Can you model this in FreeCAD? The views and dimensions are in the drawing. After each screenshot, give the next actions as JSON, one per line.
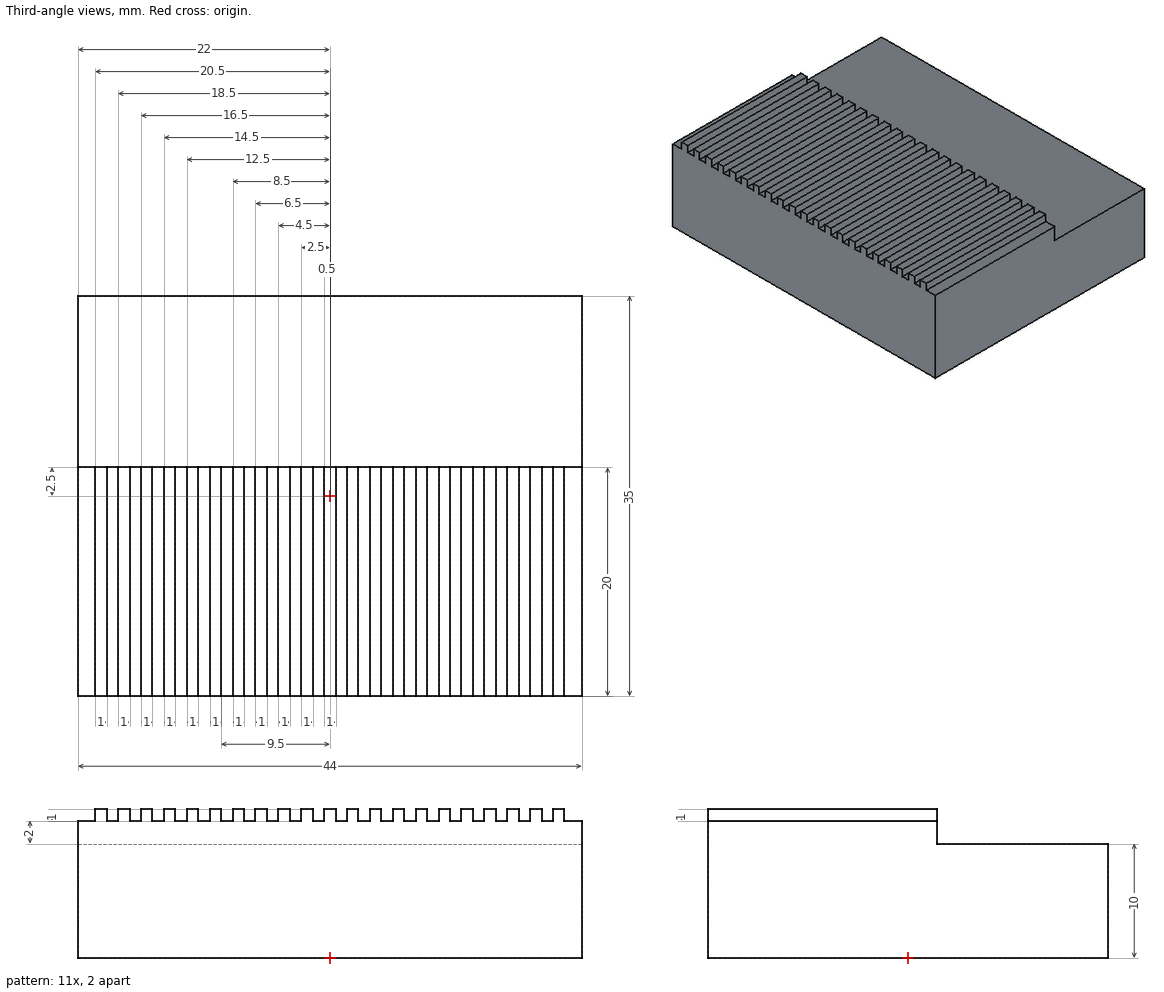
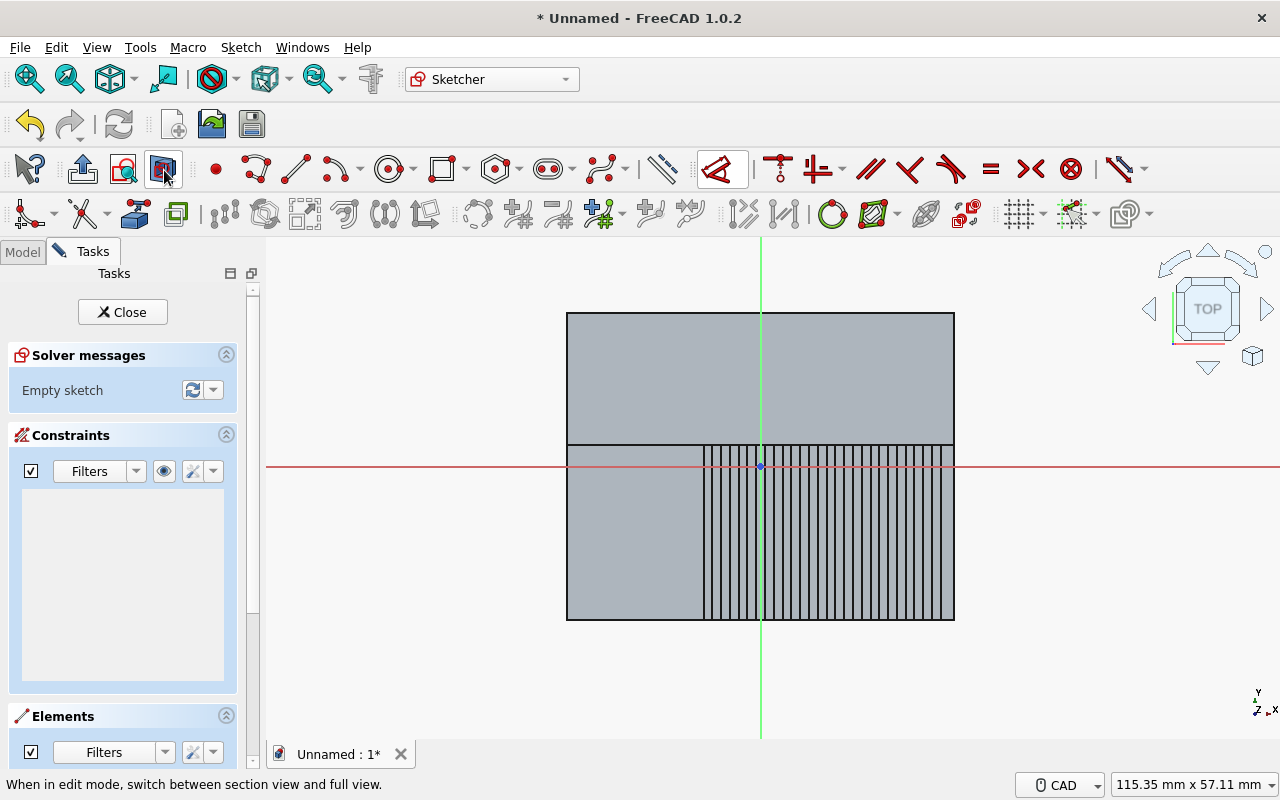
{"action": "scroll", "coordinate": [746, 587], "scroll_direction": "up", "scroll_amount": 3}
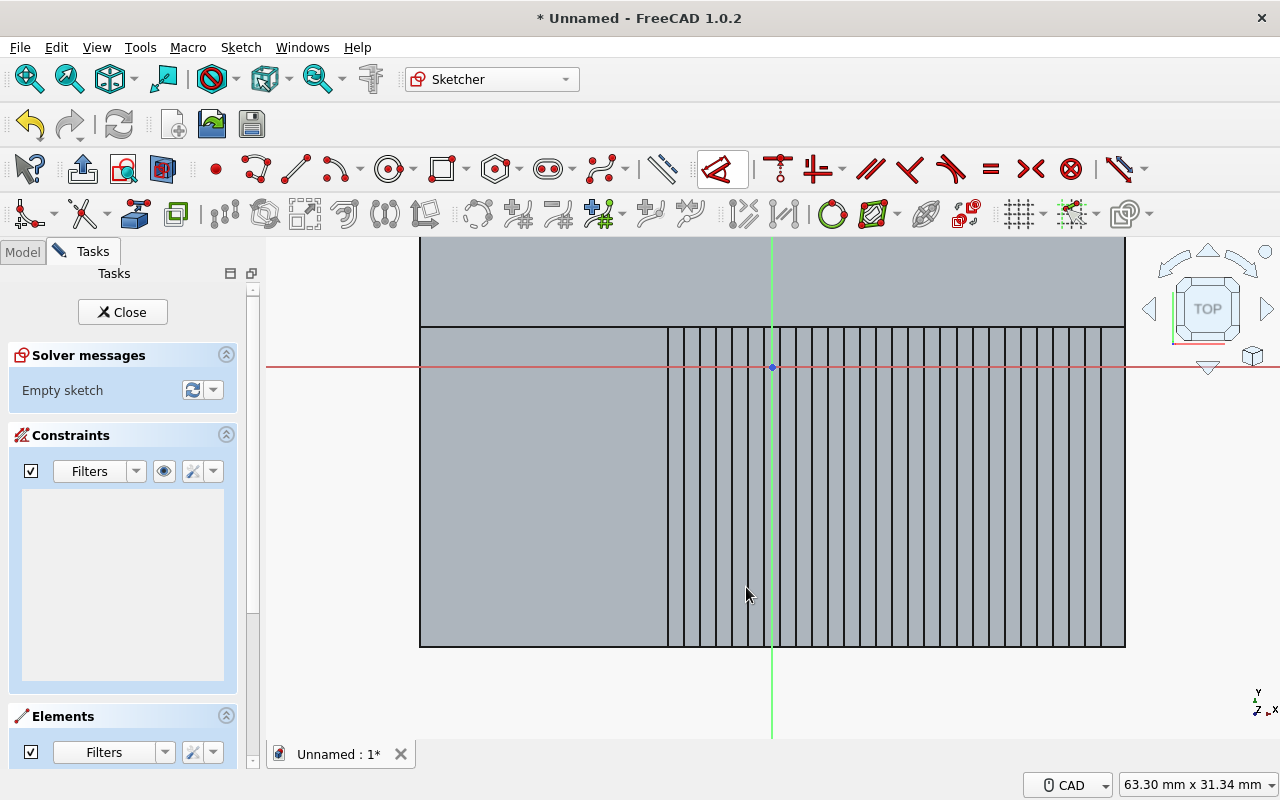
{"action": "left_click", "coordinate": [442, 170]}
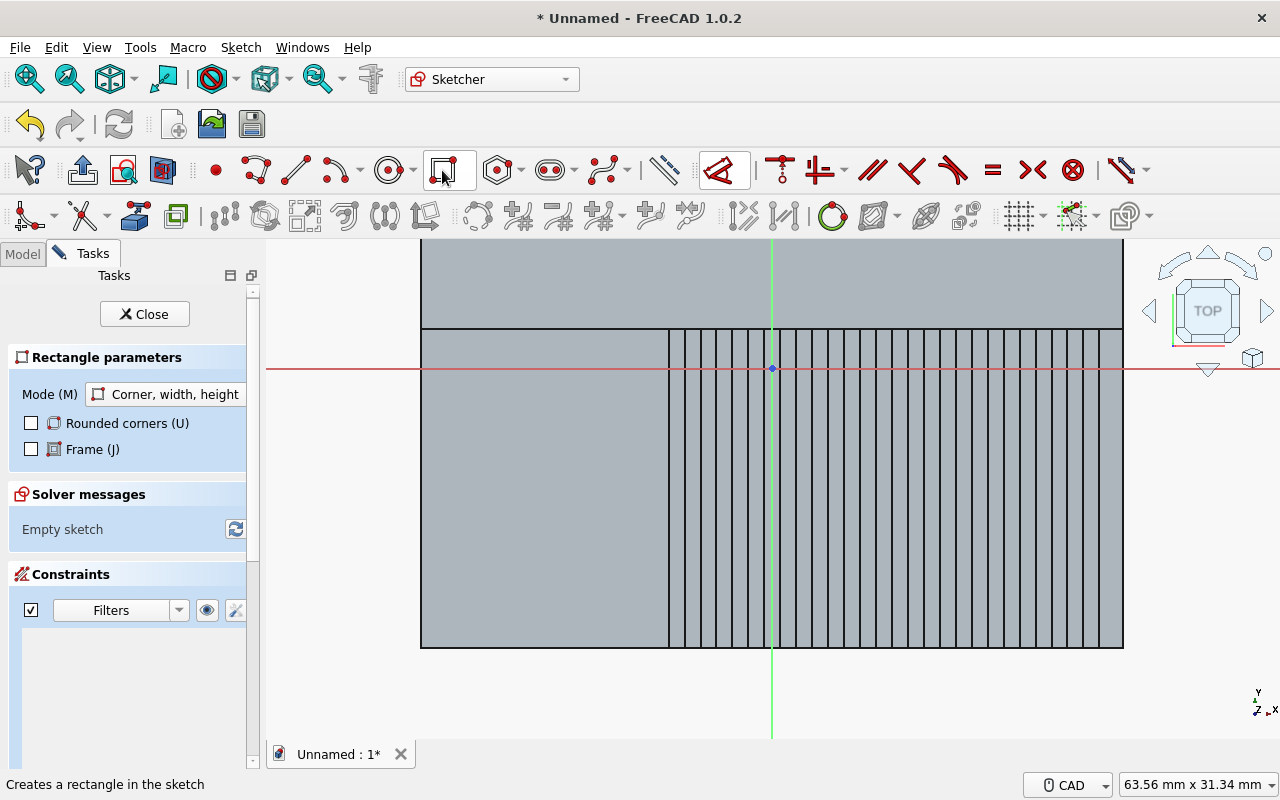
{"action": "left_click", "coordinate": [637, 329]}
{"action": "mouse_move", "coordinate": [653, 648]}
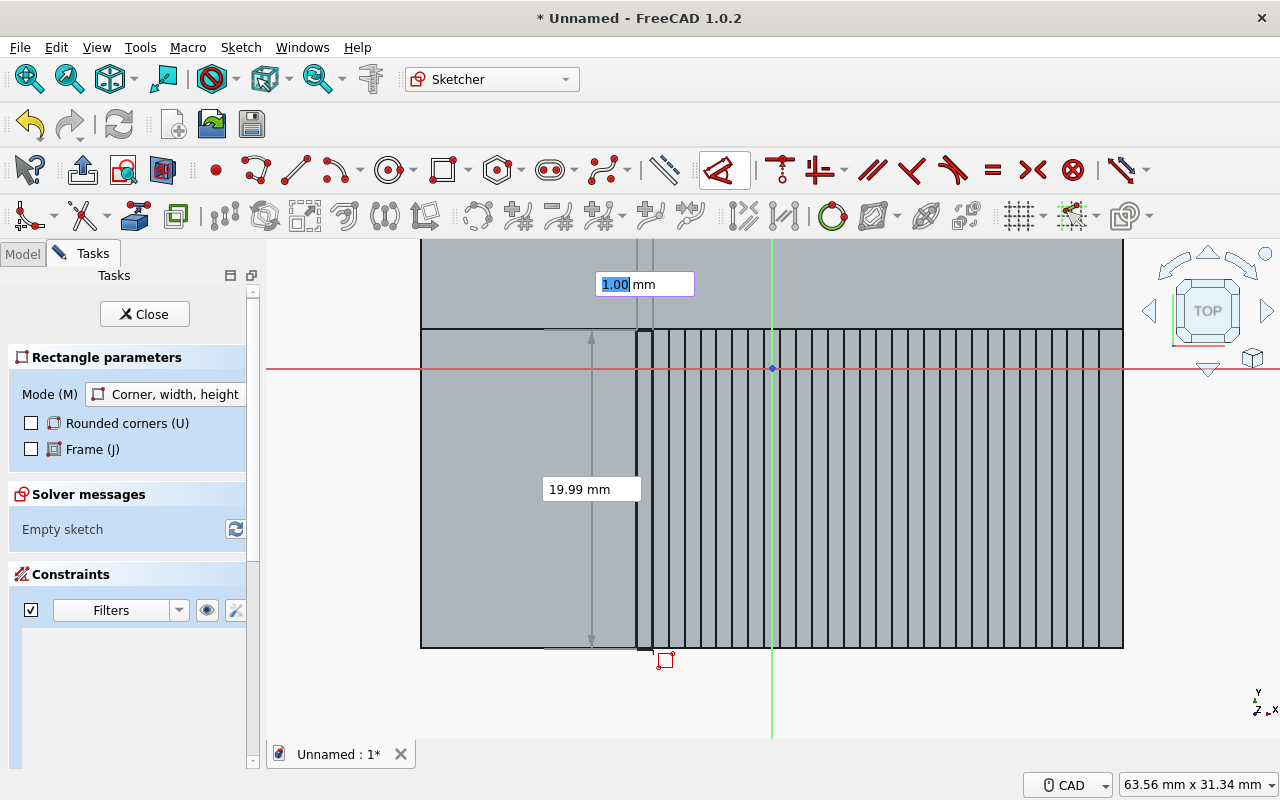
{"action": "type", "text": "1"}
{"action": "key", "text": "Tab"}
{"action": "type", "text": "20"}
{"action": "key", "text": "Return"}
{"action": "key", "text": "Escape"}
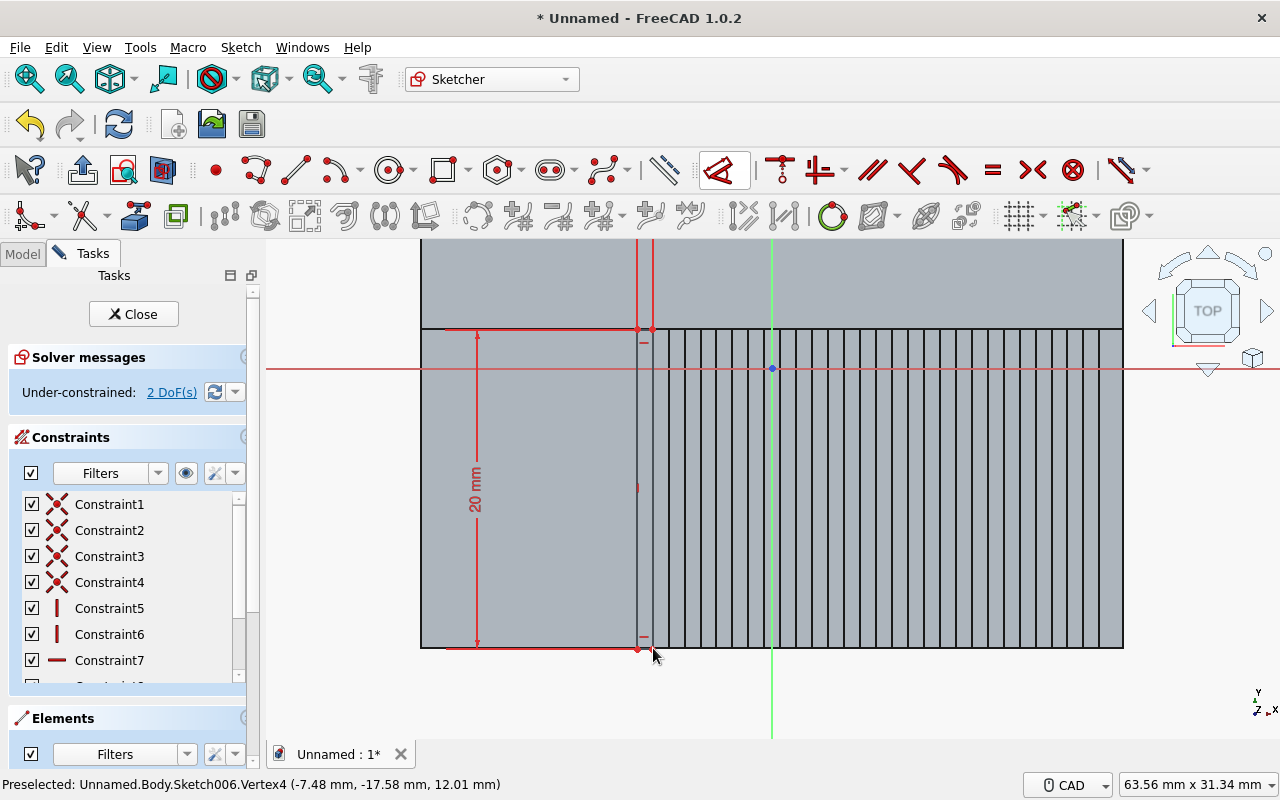
{"action": "left_click", "coordinate": [637, 330]}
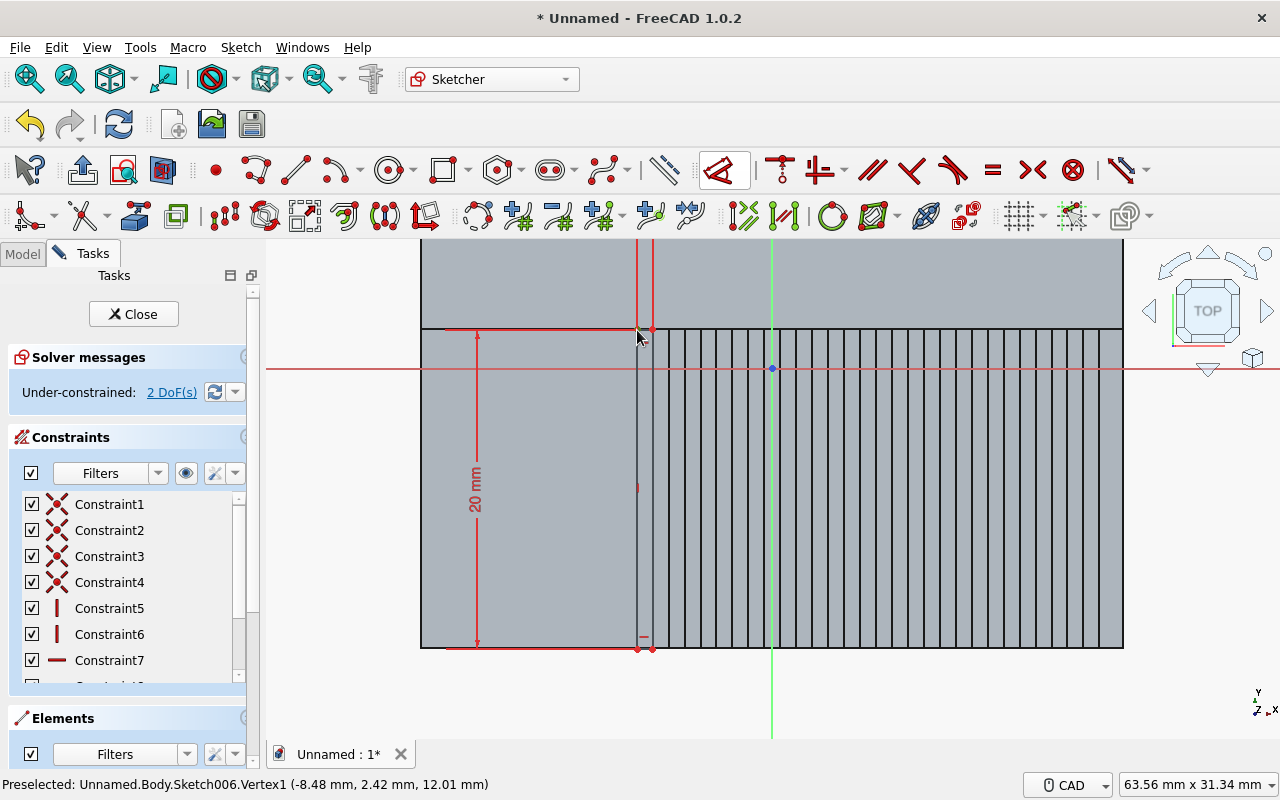
{"action": "left_click", "coordinate": [744, 170]}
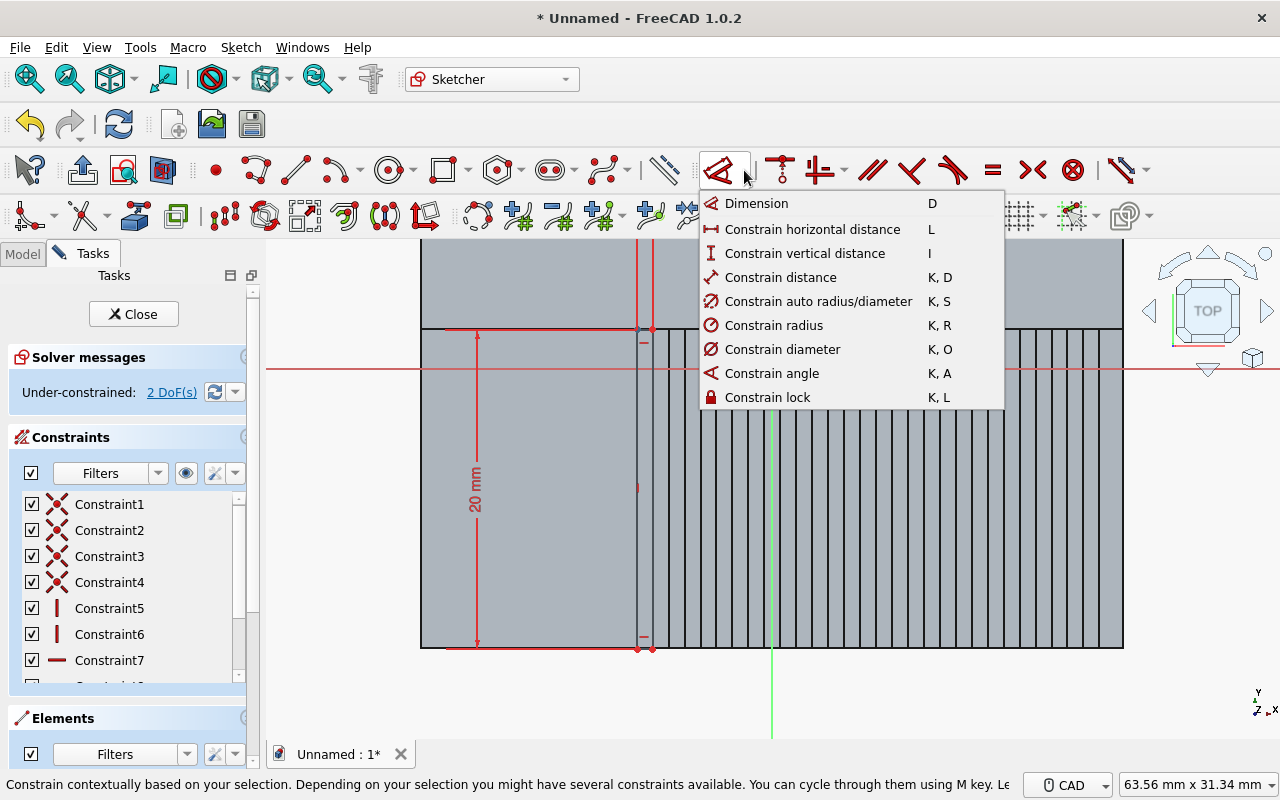
{"action": "left_click", "coordinate": [852, 229]}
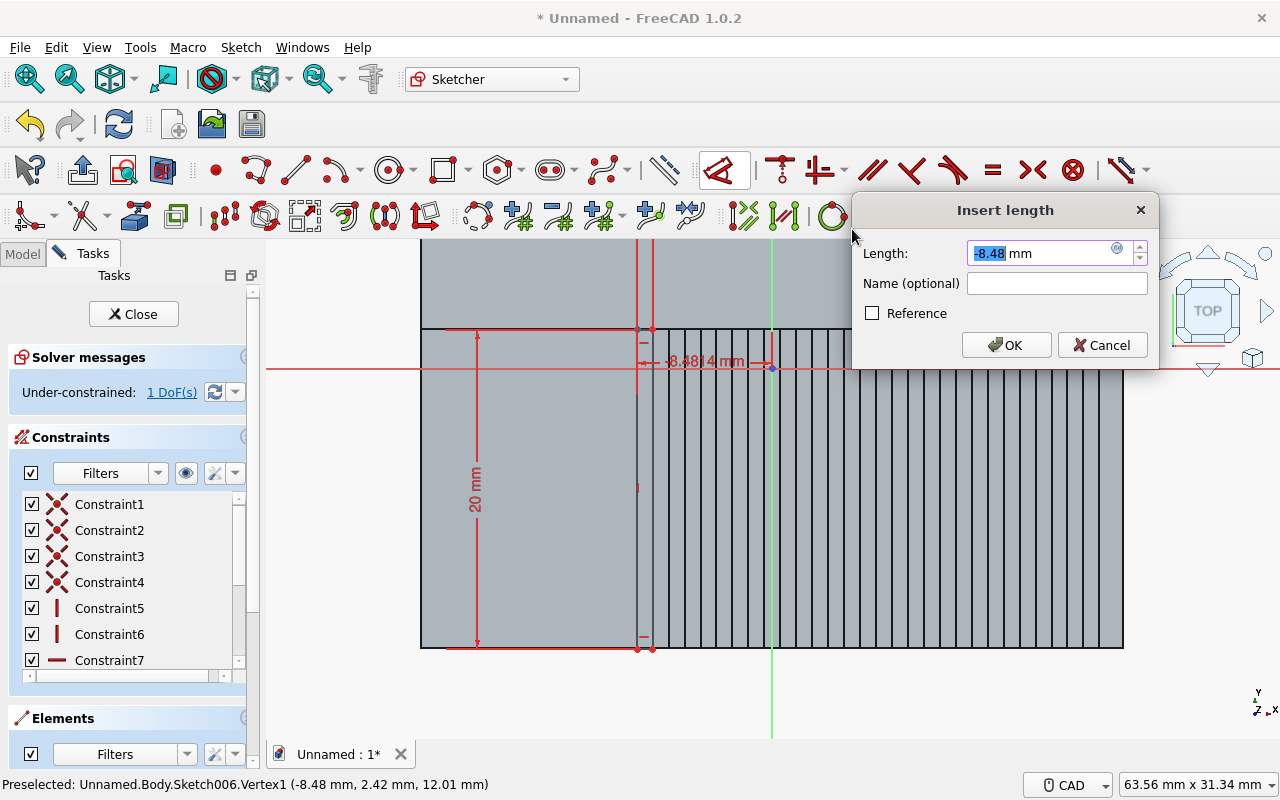
{"action": "type", "text": "-8.5"}
{"action": "key", "text": "Return"}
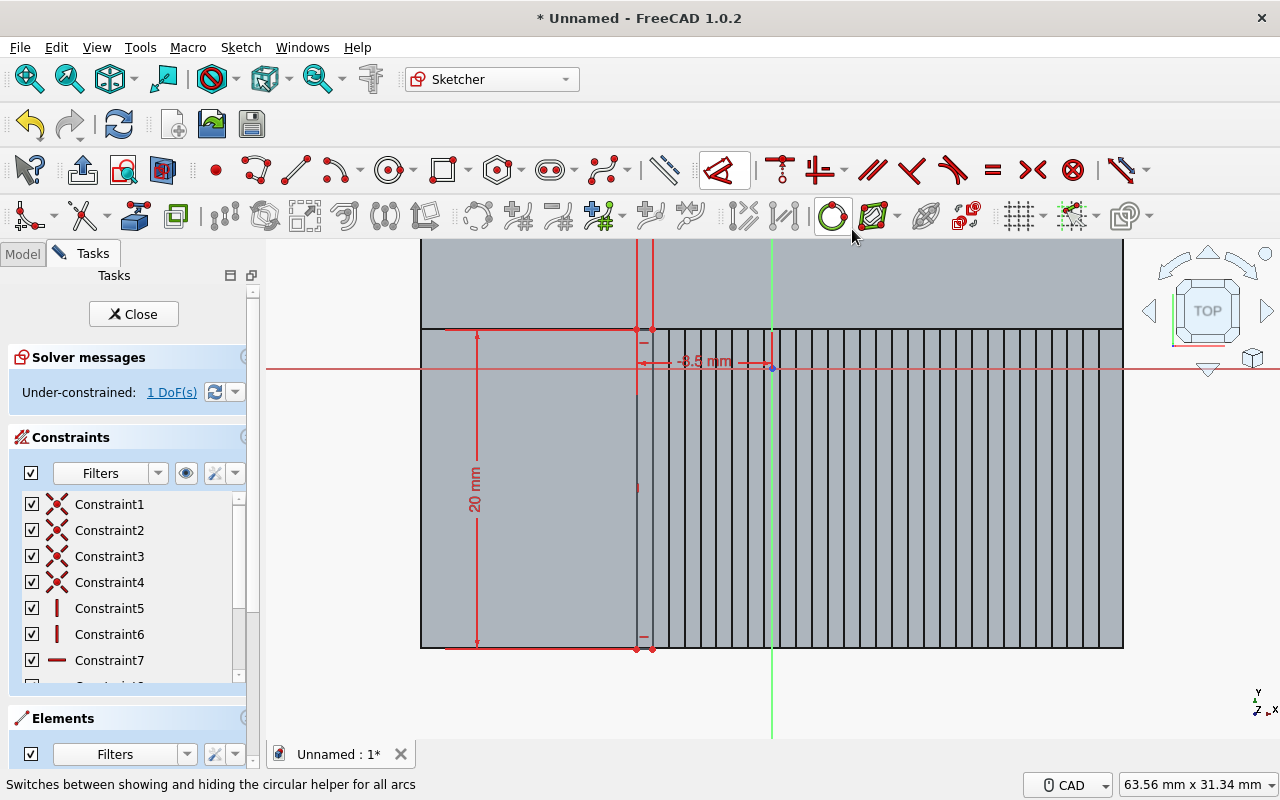
{"action": "left_click", "coordinate": [637, 330]}